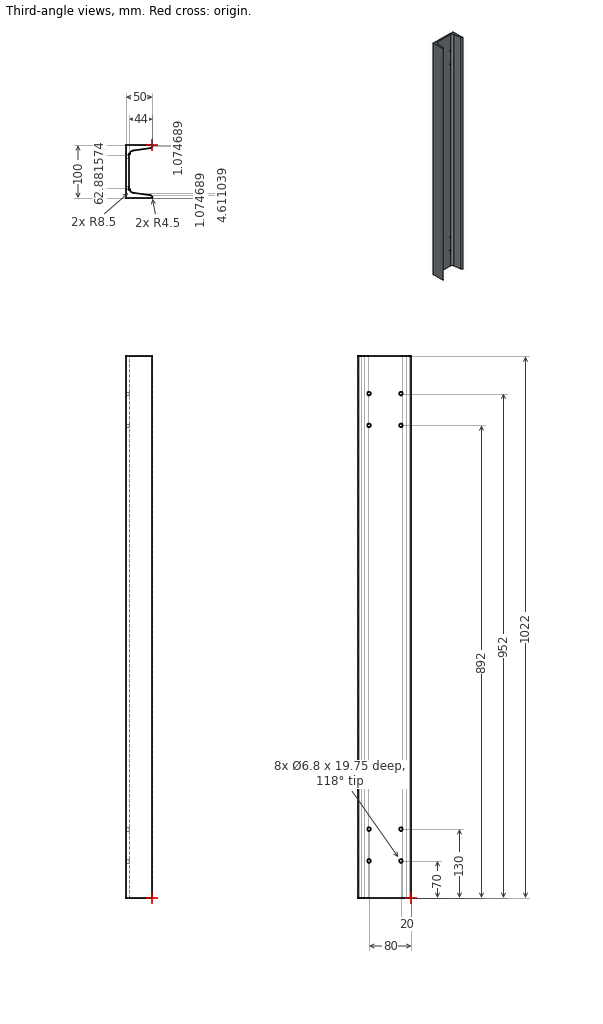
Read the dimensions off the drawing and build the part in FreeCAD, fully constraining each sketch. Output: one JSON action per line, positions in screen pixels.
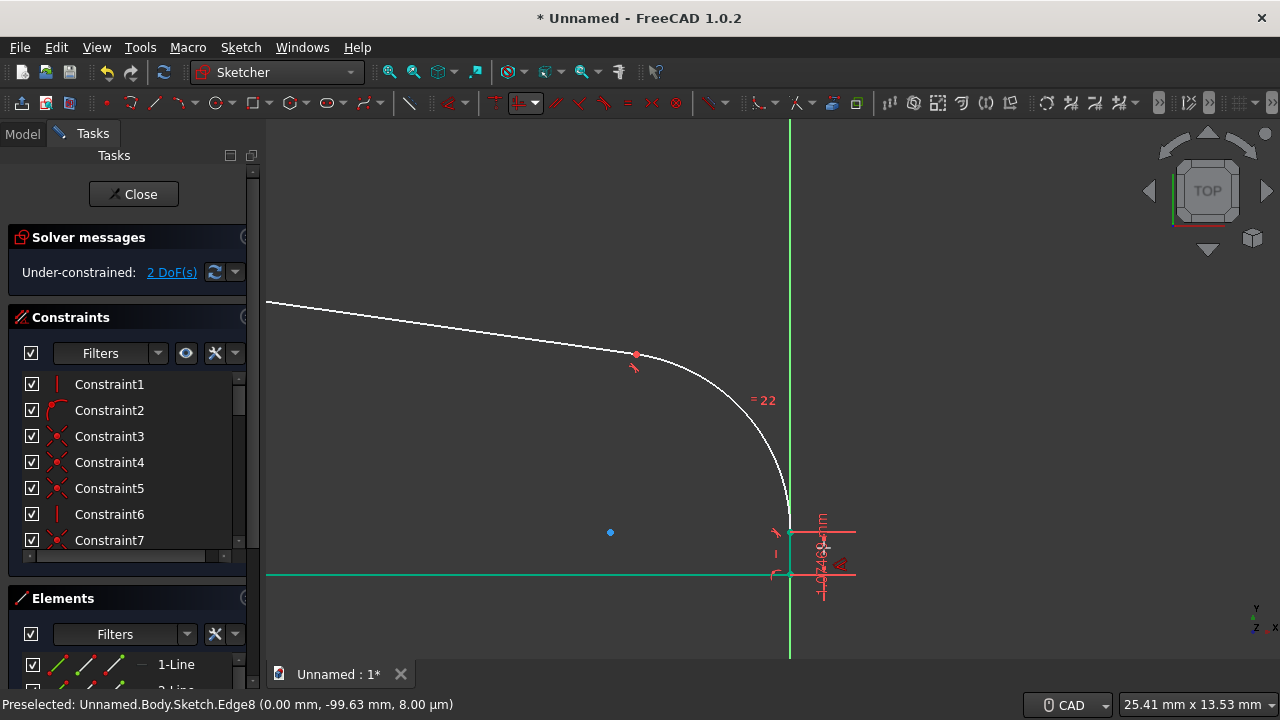
{"action": "scroll", "coordinate": [795, 569], "scroll_direction": "down", "scroll_amount": 12}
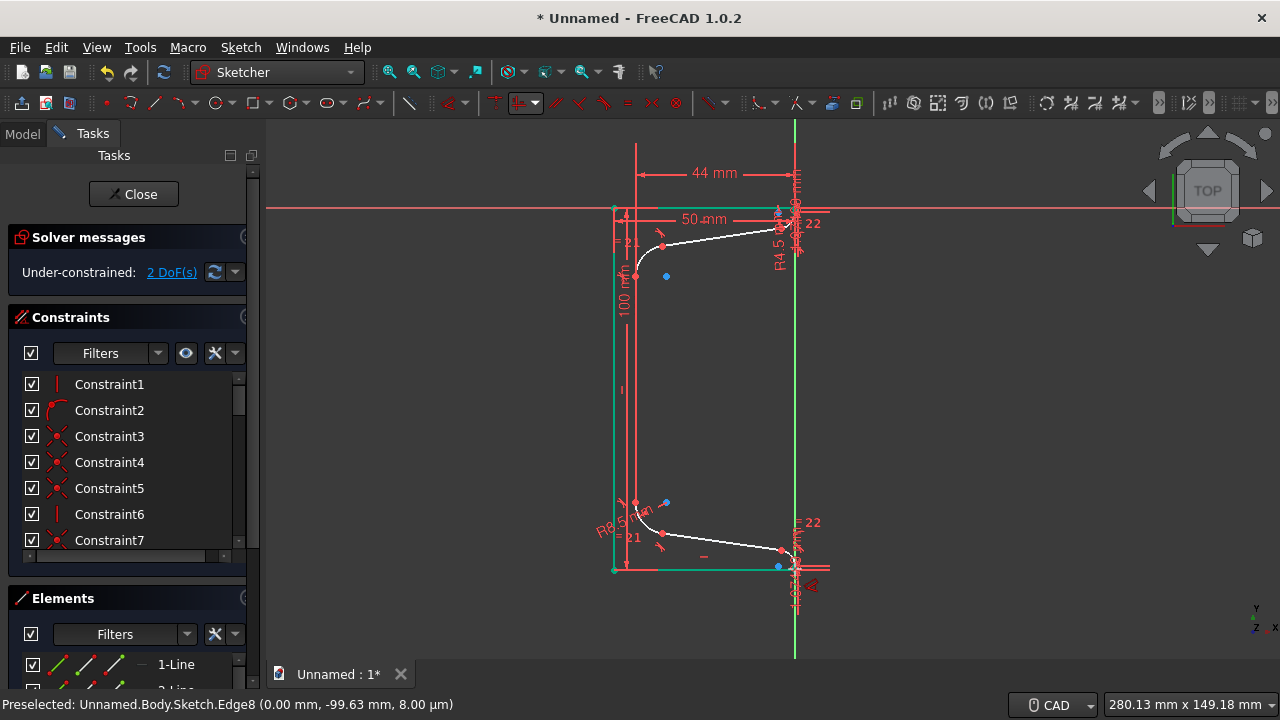
{"action": "left_click", "coordinate": [636, 435]}
{"action": "left_click", "coordinate": [670, 390]}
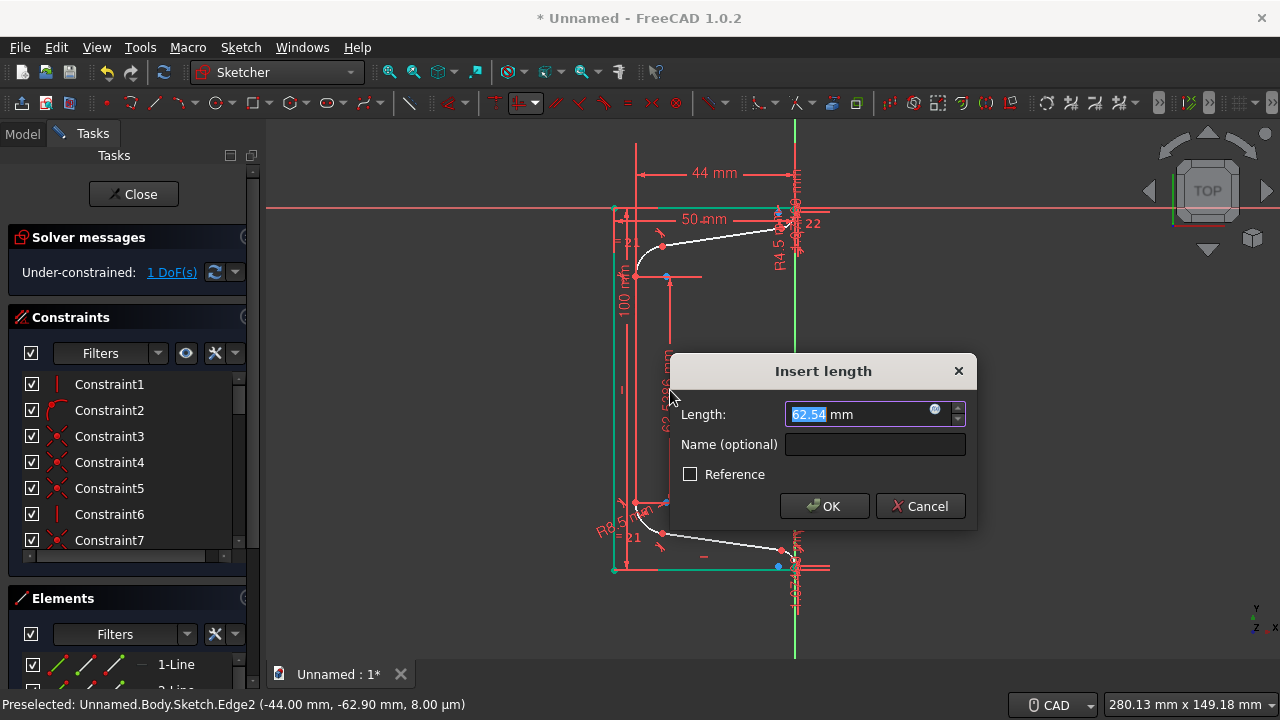
{"action": "type", "text": "62.881574"}
{"action": "key", "text": "Return"}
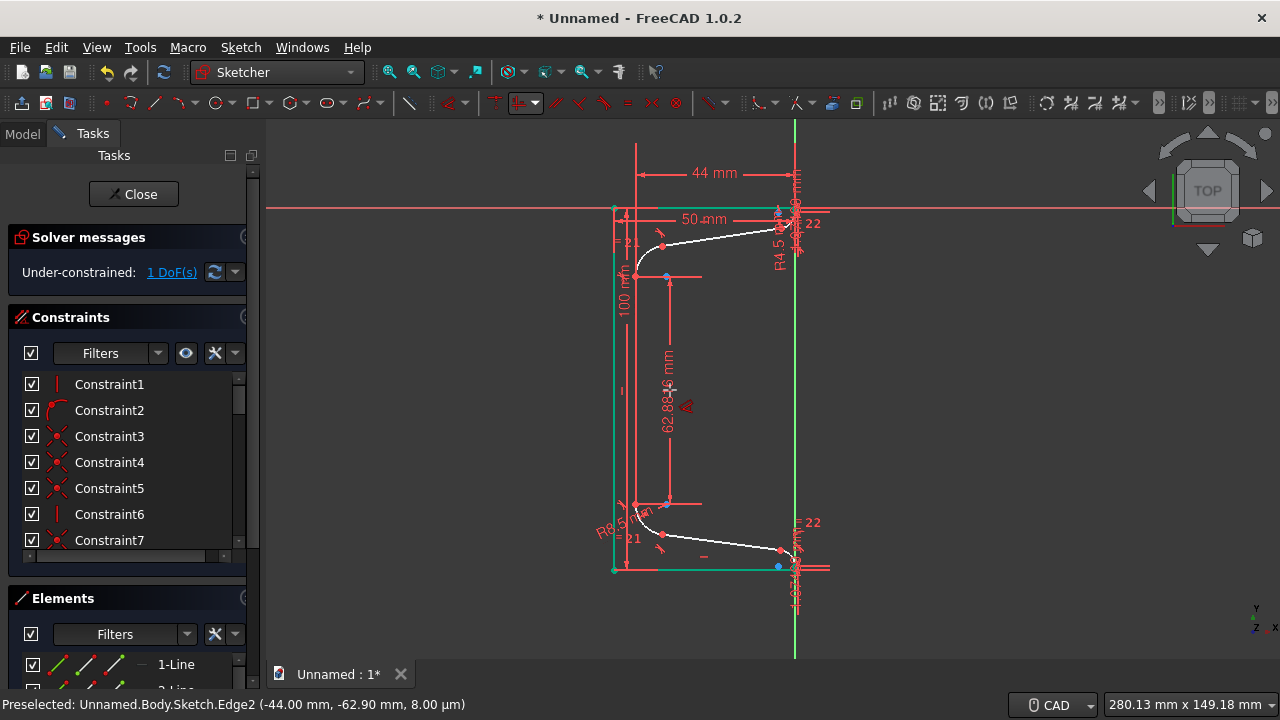
{"action": "scroll", "coordinate": [745, 546], "scroll_direction": "up", "scroll_amount": 5}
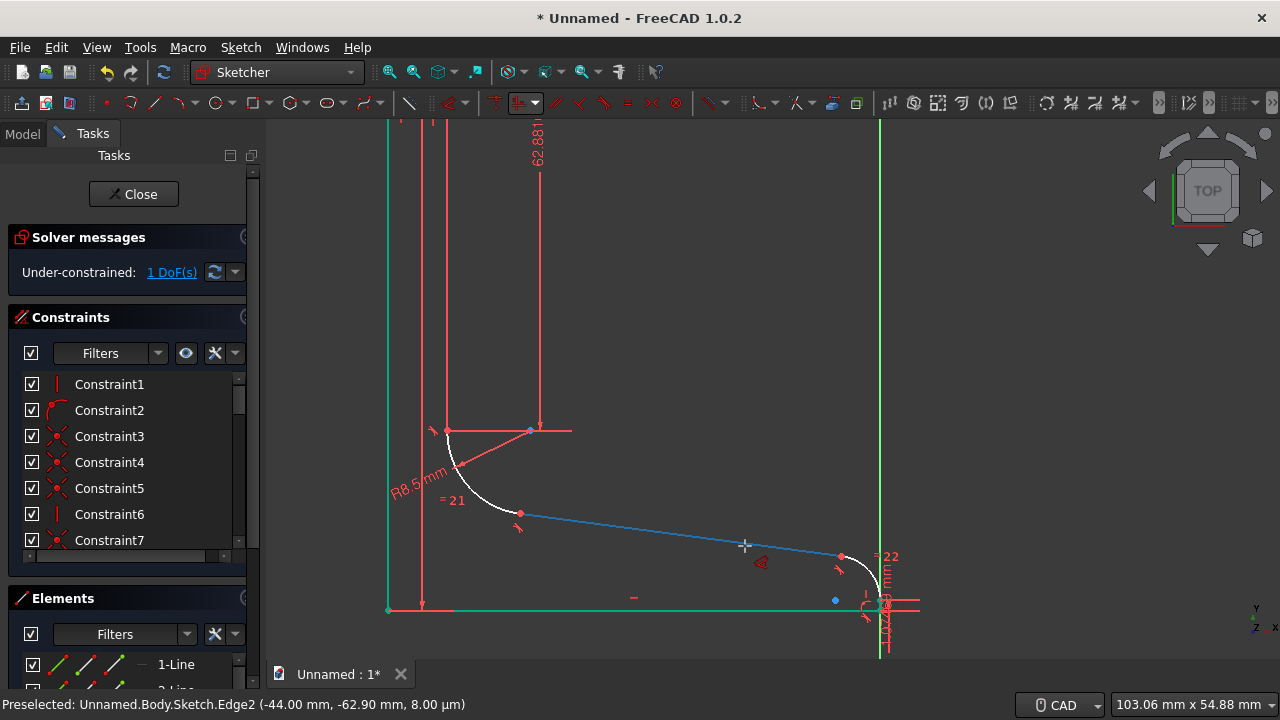
{"action": "left_click", "coordinate": [745, 543]}
{"action": "left_click", "coordinate": [486, 535]}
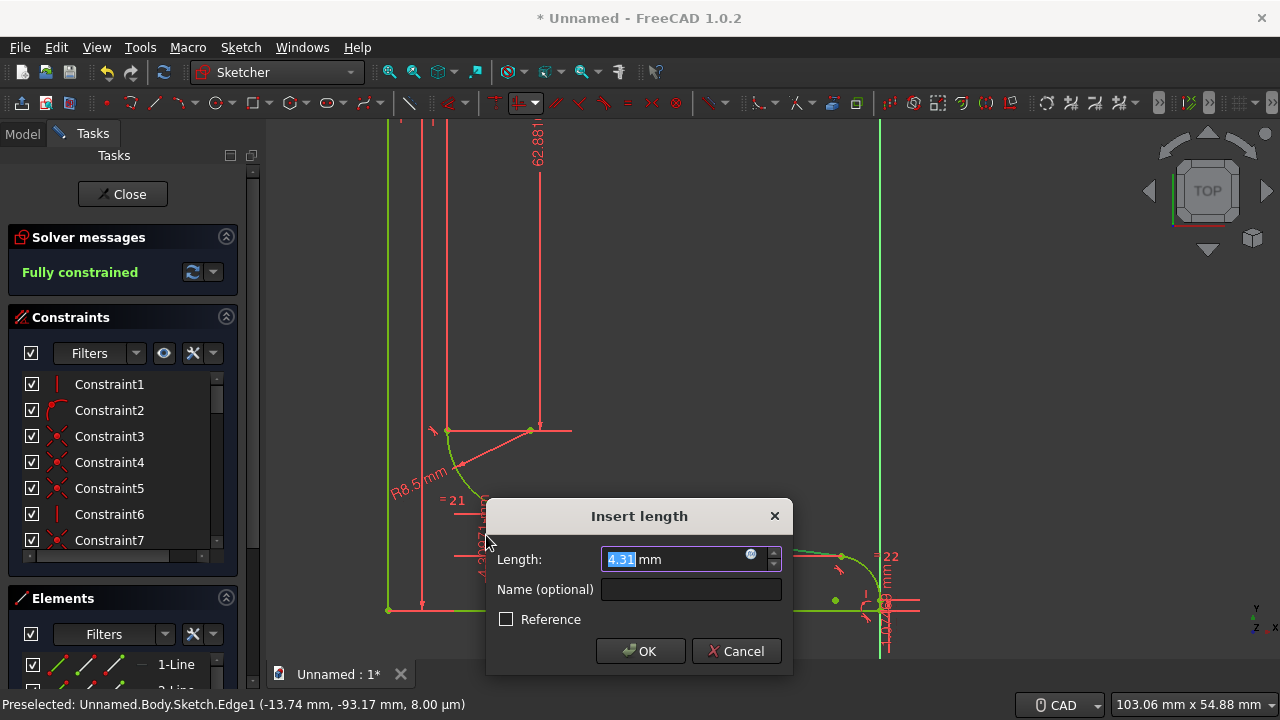
{"action": "type", "text": "4.611039"}
{"action": "key", "text": "Return"}
{"action": "key", "text": "Escape"}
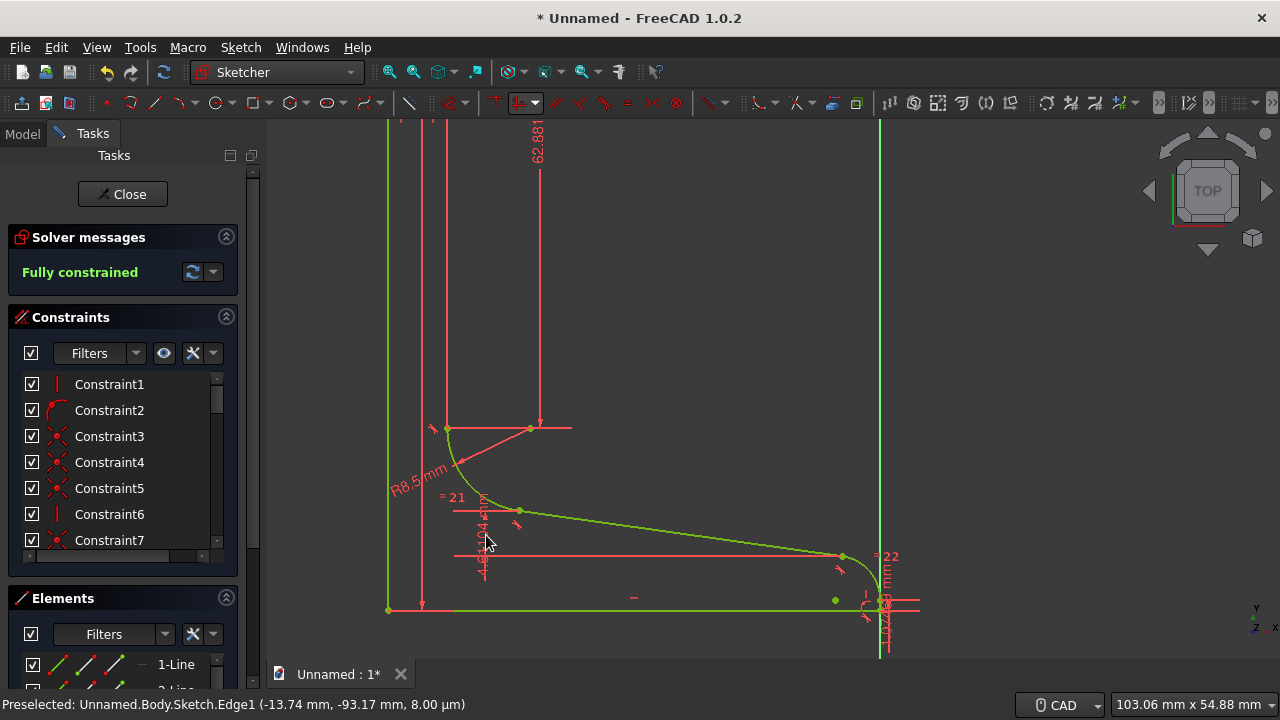
{"action": "left_click", "coordinate": [123, 194]}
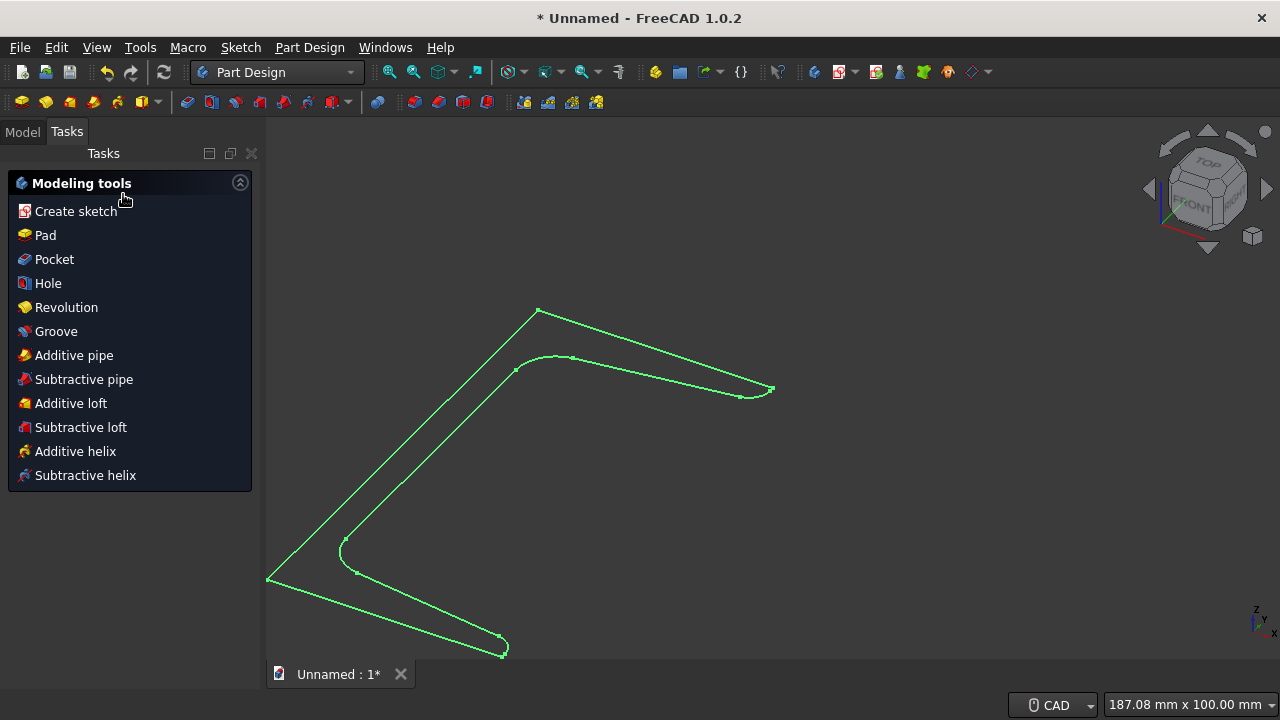
{"action": "left_click", "coordinate": [22, 102]}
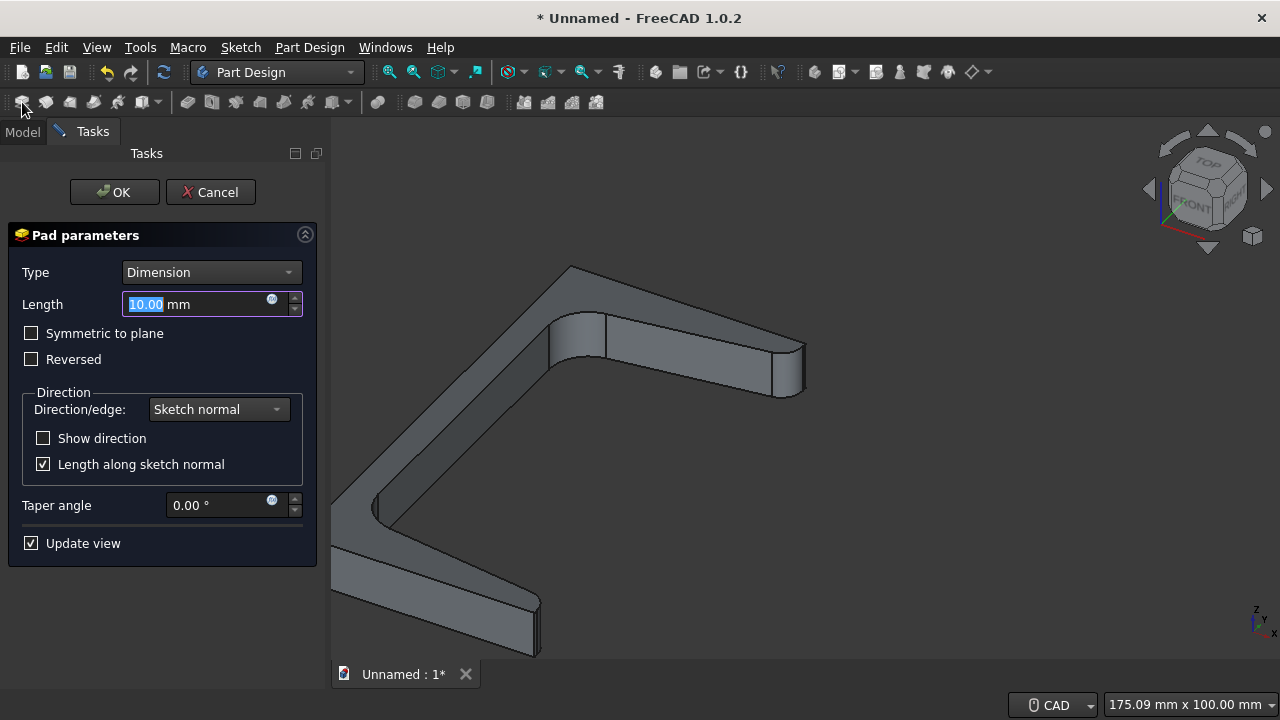
{"action": "type", "text": "1022"}
{"action": "key", "text": "Tab"}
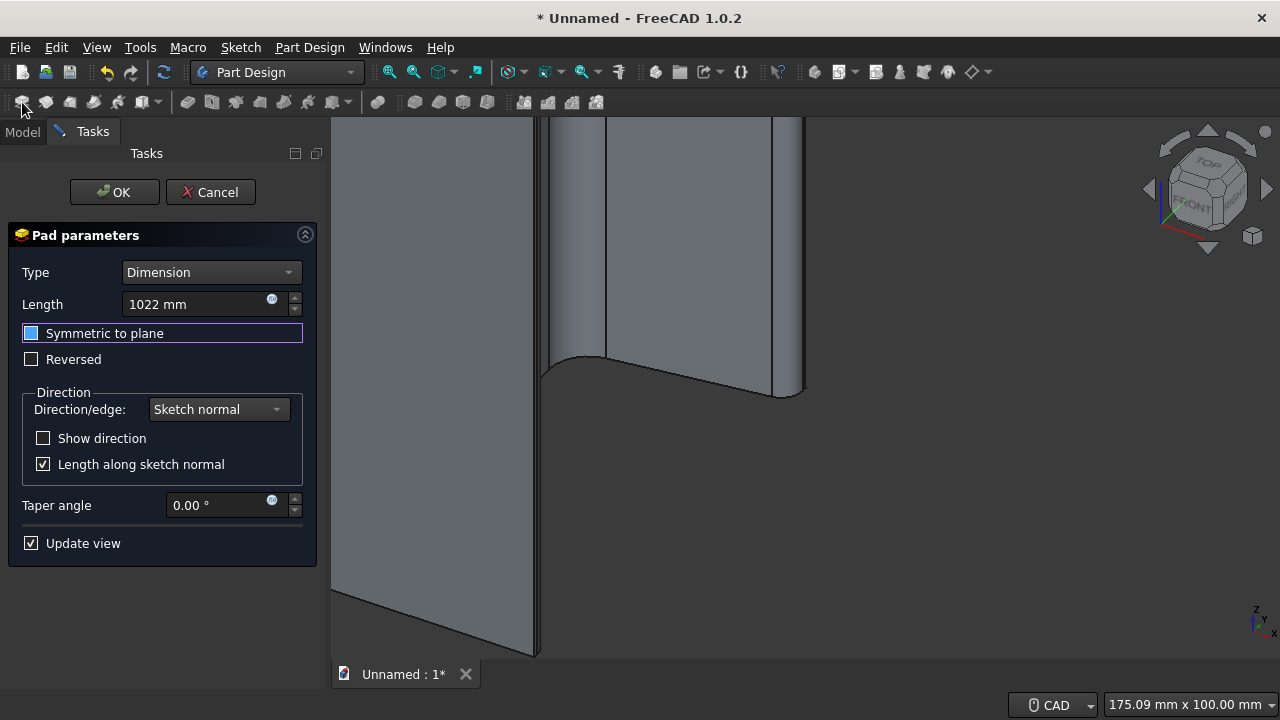
{"action": "left_click", "coordinate": [115, 192]}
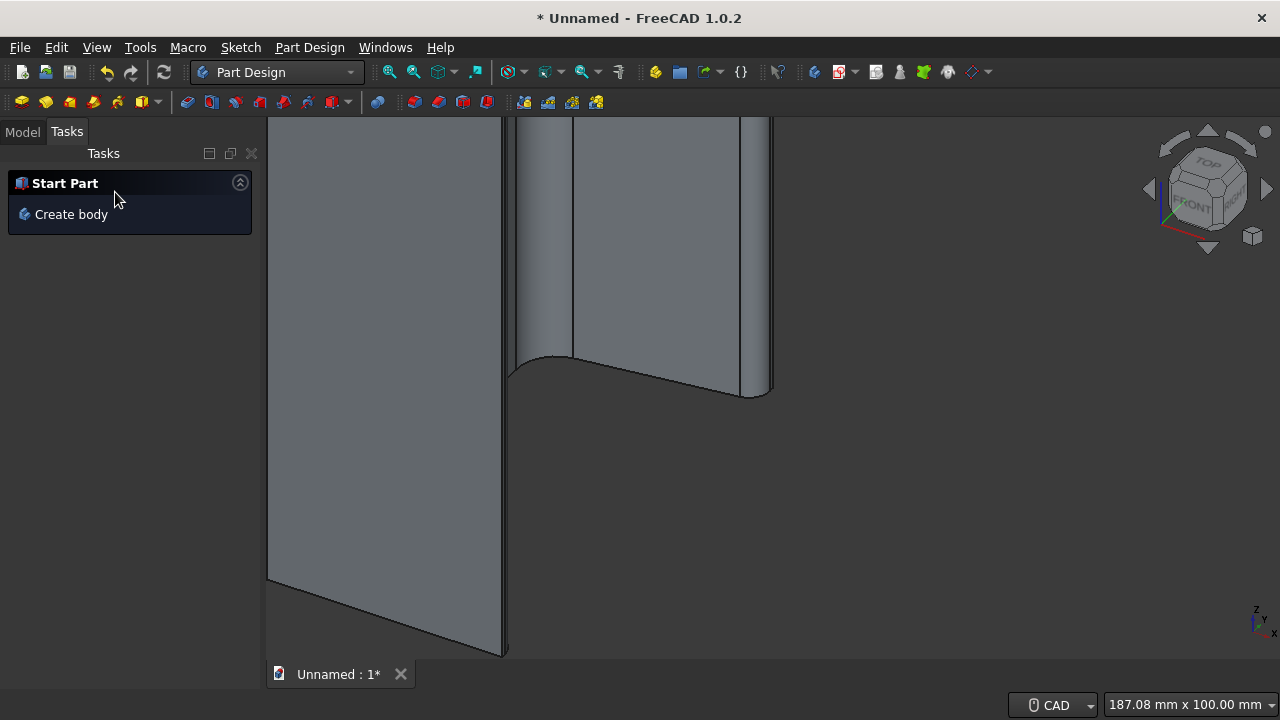
{"action": "left_click", "coordinate": [390, 72]}